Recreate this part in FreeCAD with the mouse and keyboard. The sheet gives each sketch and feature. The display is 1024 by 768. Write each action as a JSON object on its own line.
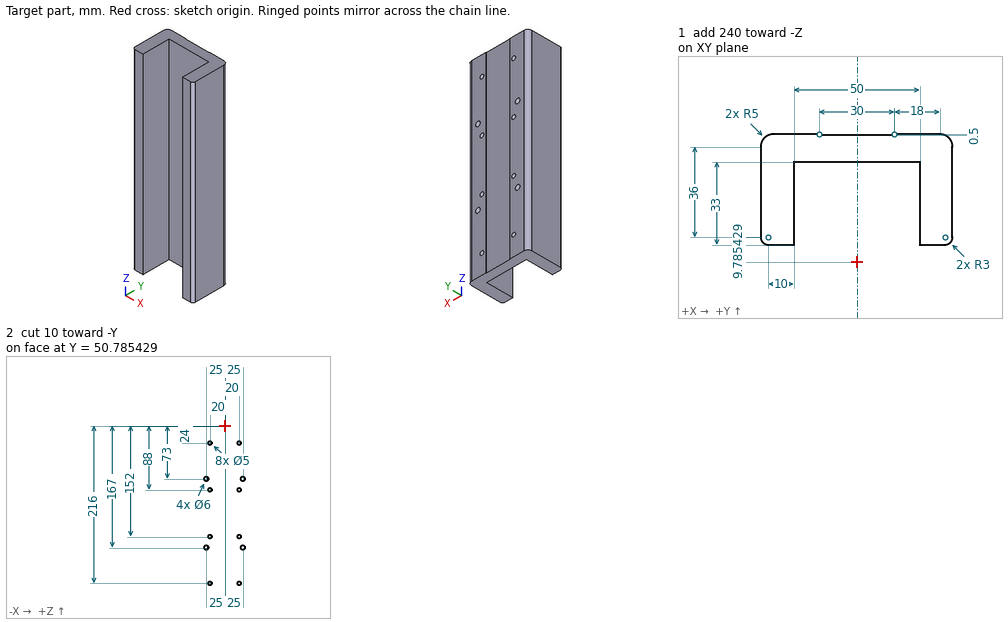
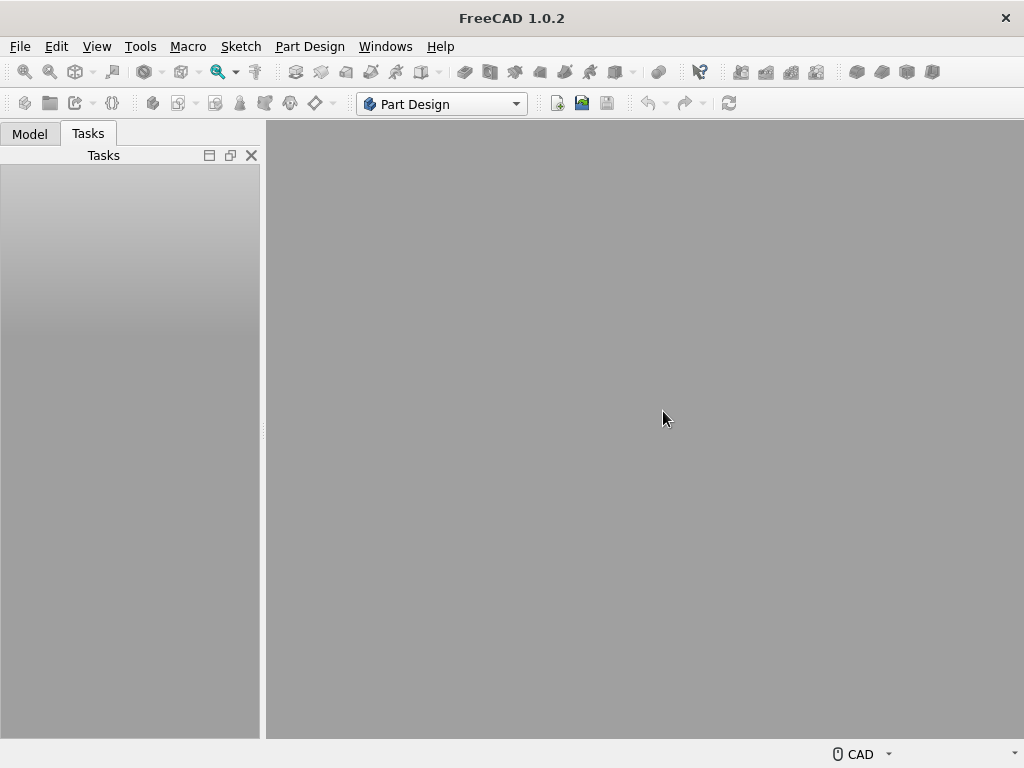
{"action": "left_click", "coordinate": [557, 104]}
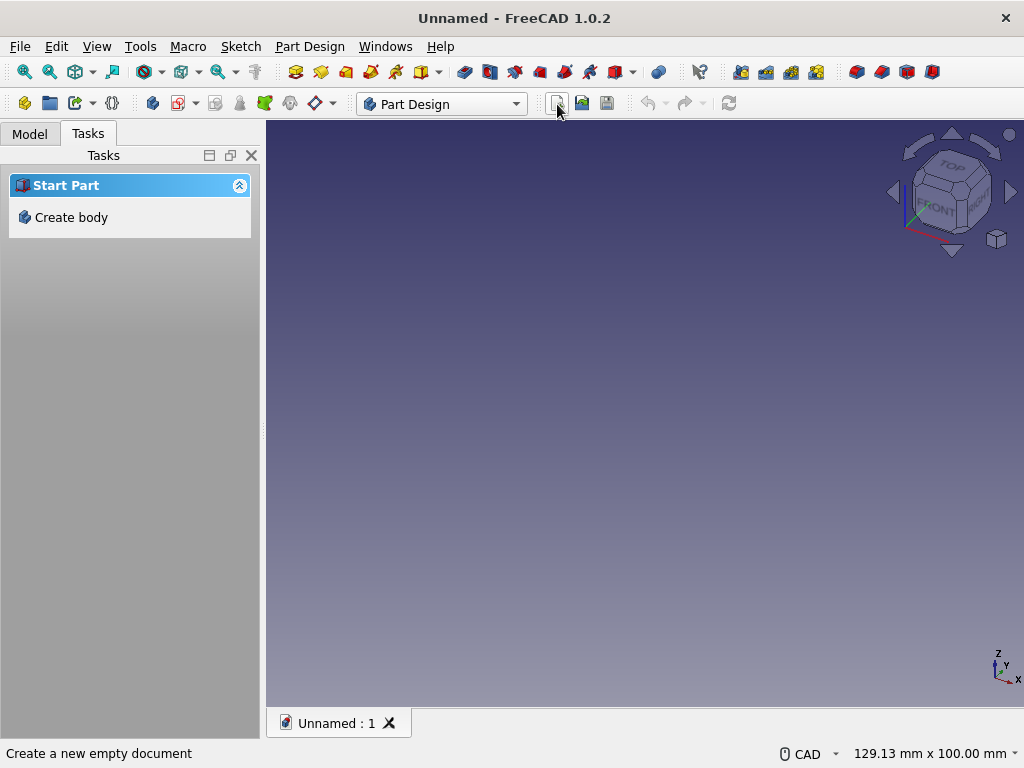
{"action": "left_click", "coordinate": [178, 104]}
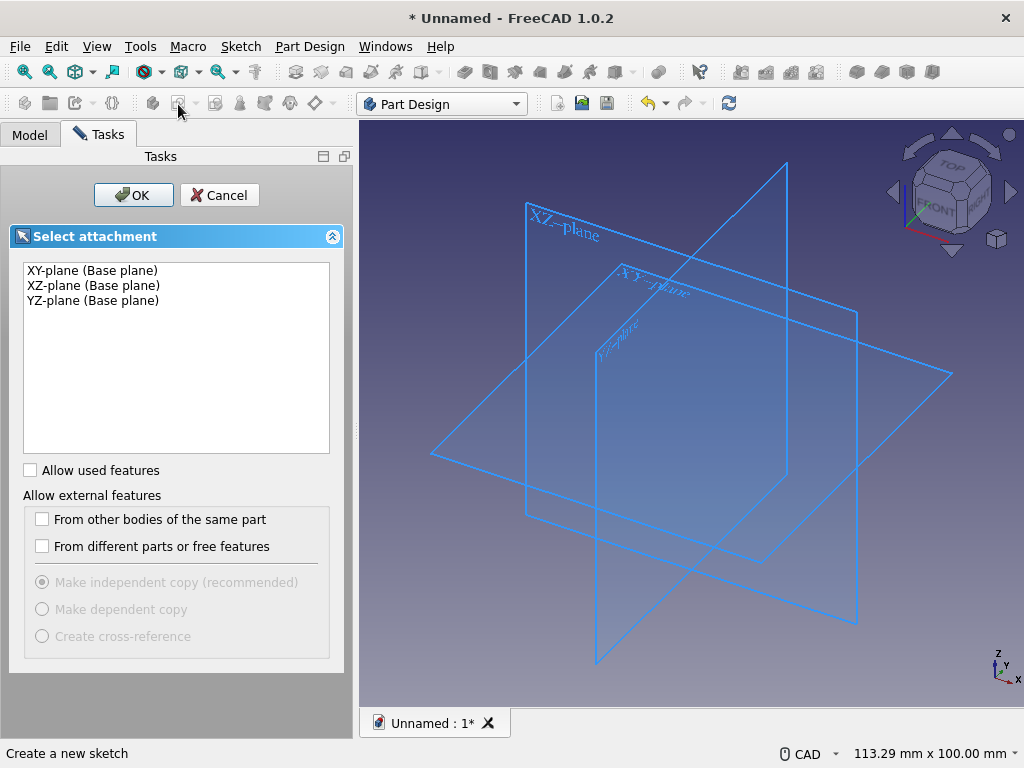
{"action": "left_click", "coordinate": [84, 270]}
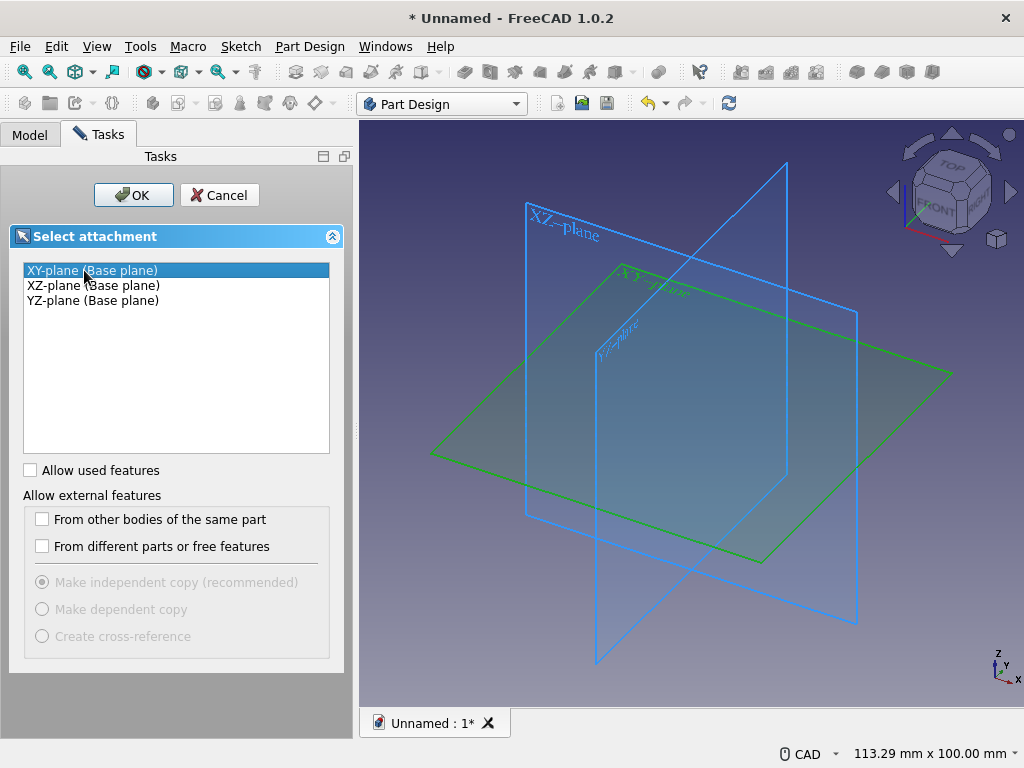
{"action": "left_click", "coordinate": [134, 195]}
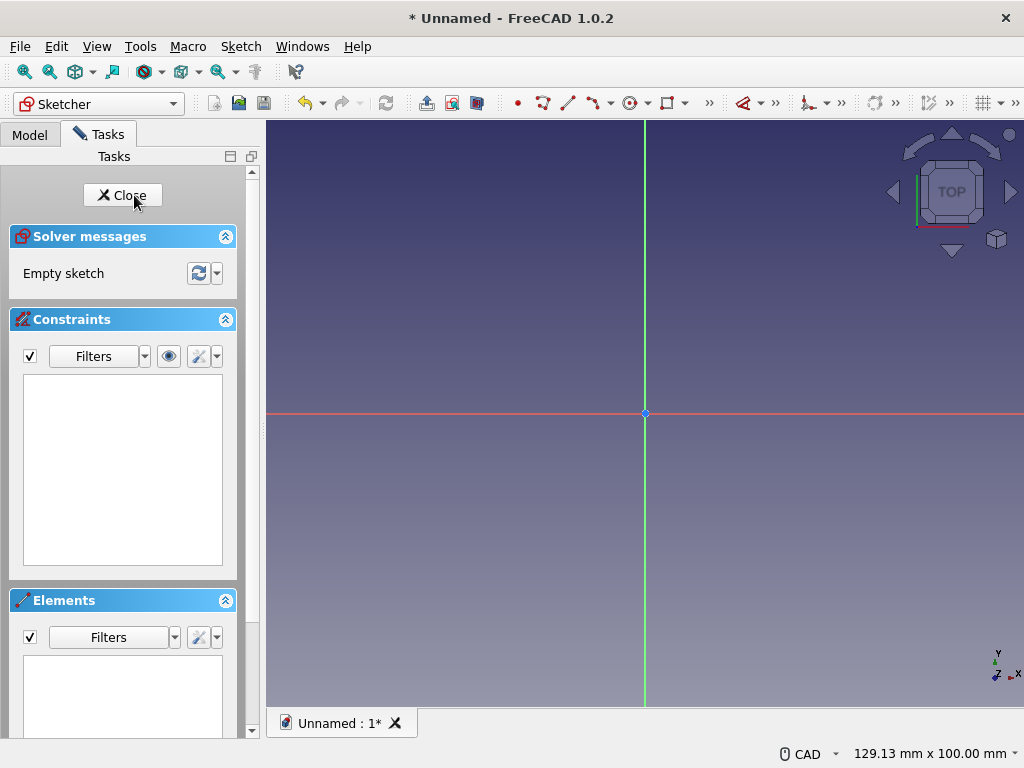
{"action": "scroll", "coordinate": [294, 679], "scroll_direction": "down", "scroll_amount": 1}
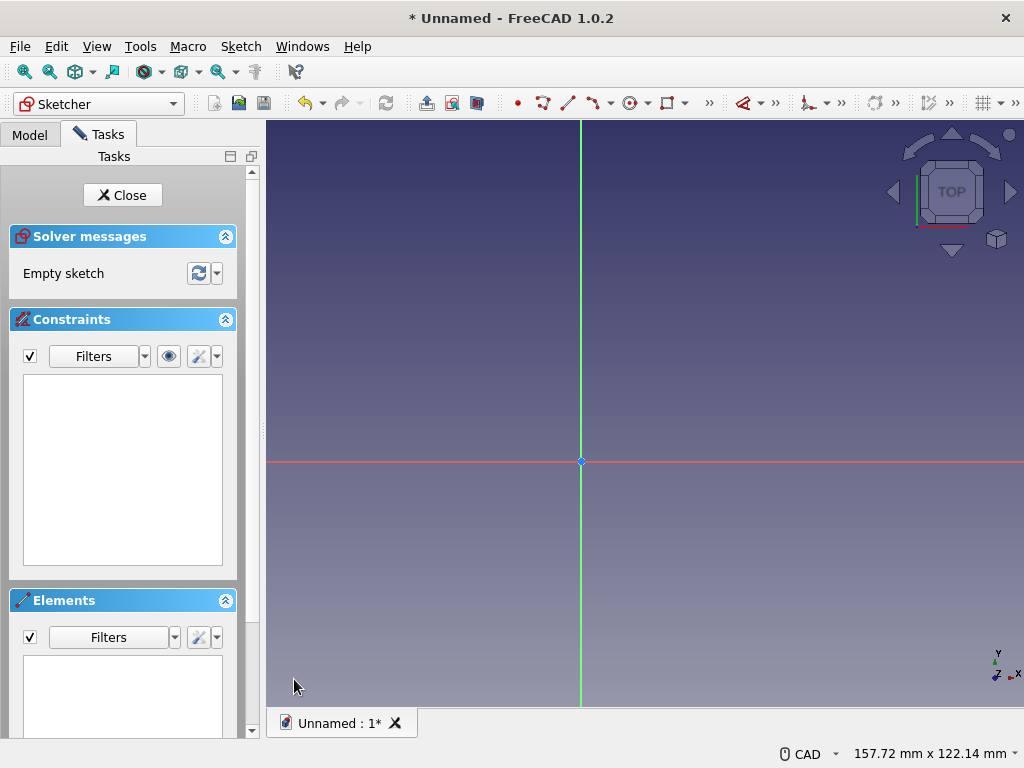
{"action": "left_click", "coordinate": [543, 104]}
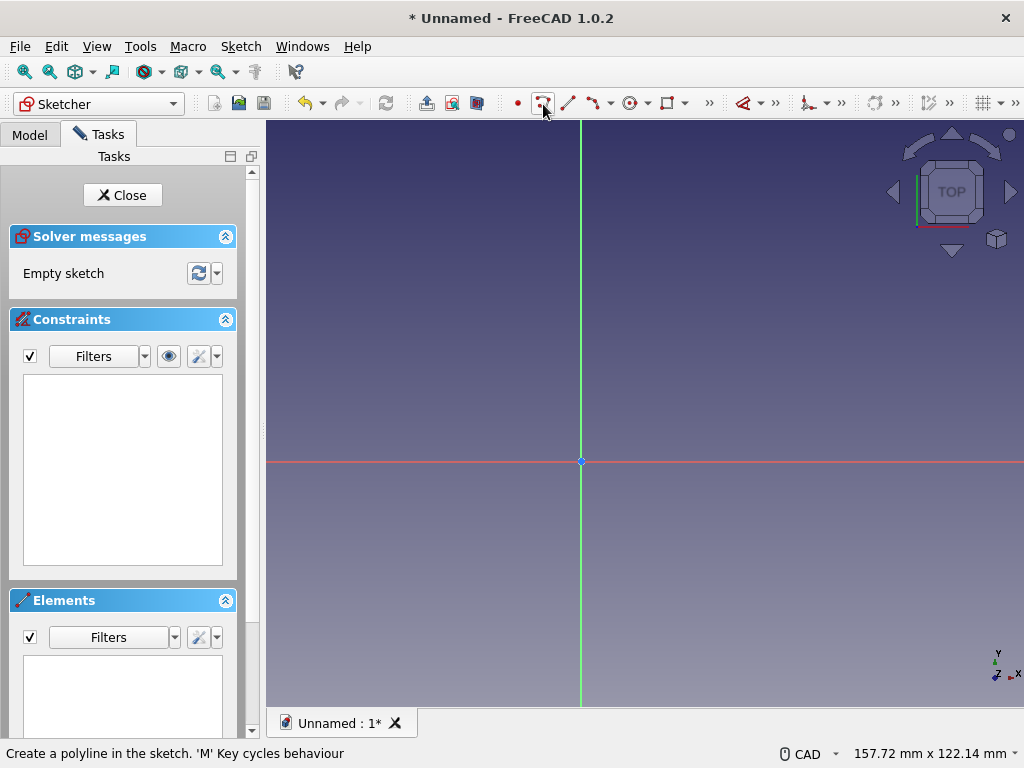
{"action": "left_click", "coordinate": [740, 218]}
{"action": "left_click", "coordinate": [653, 218]}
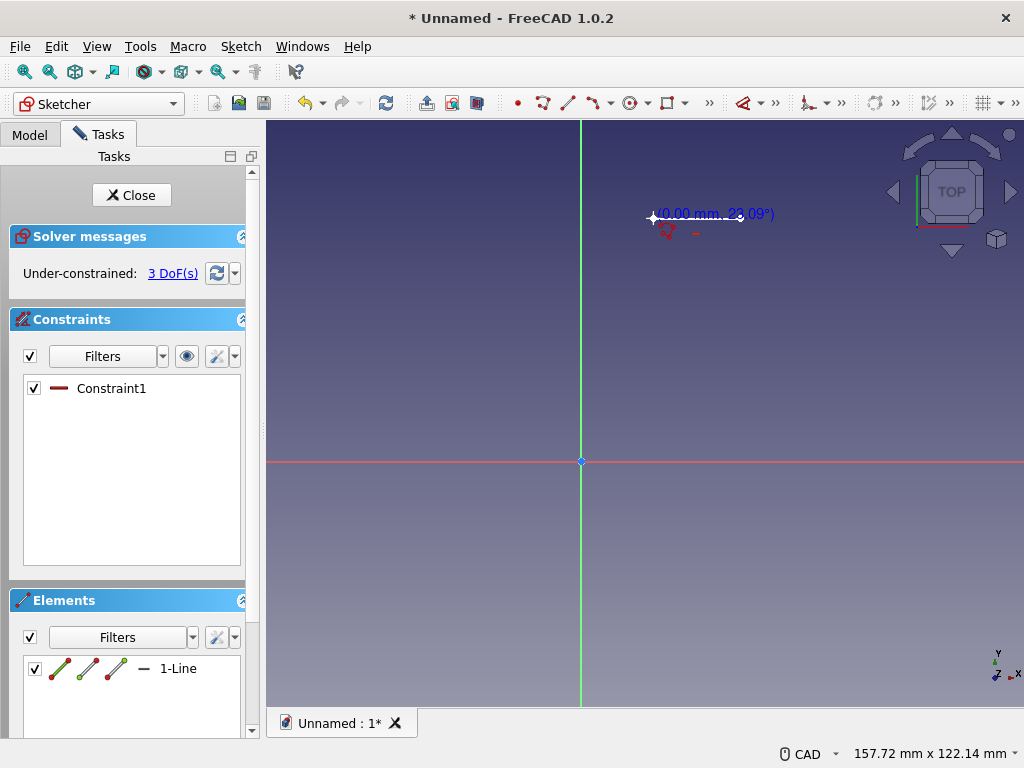
{"action": "scroll", "coordinate": [653, 220], "scroll_direction": "up", "scroll_amount": 10}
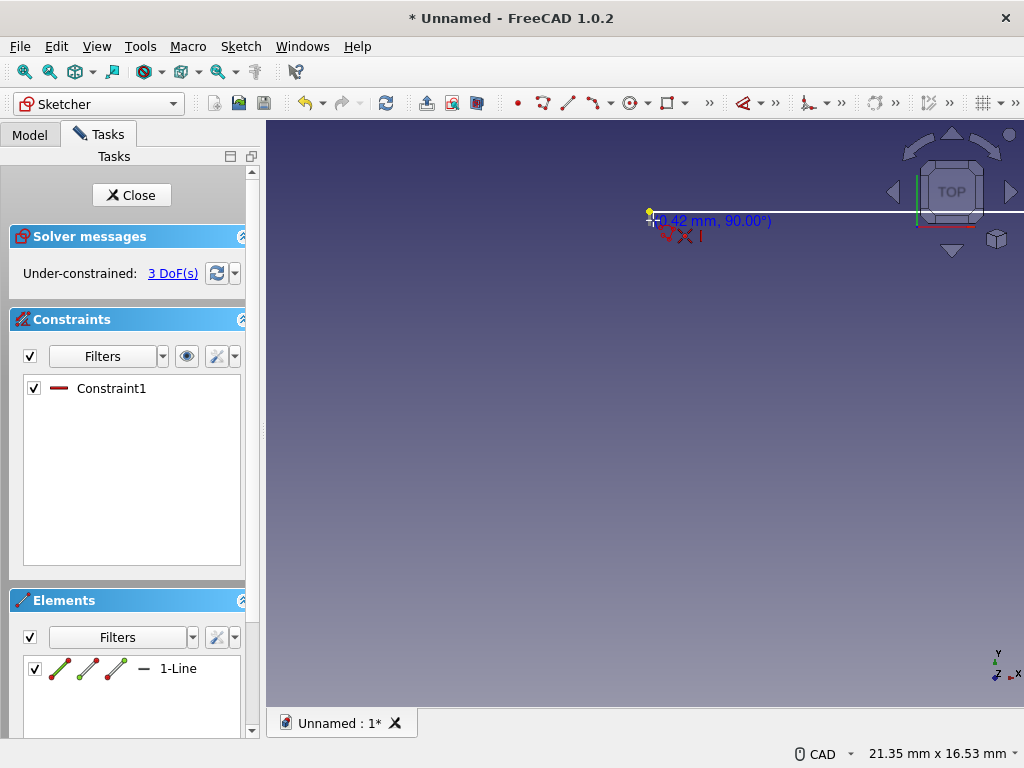
{"action": "left_click", "coordinate": [650, 220]}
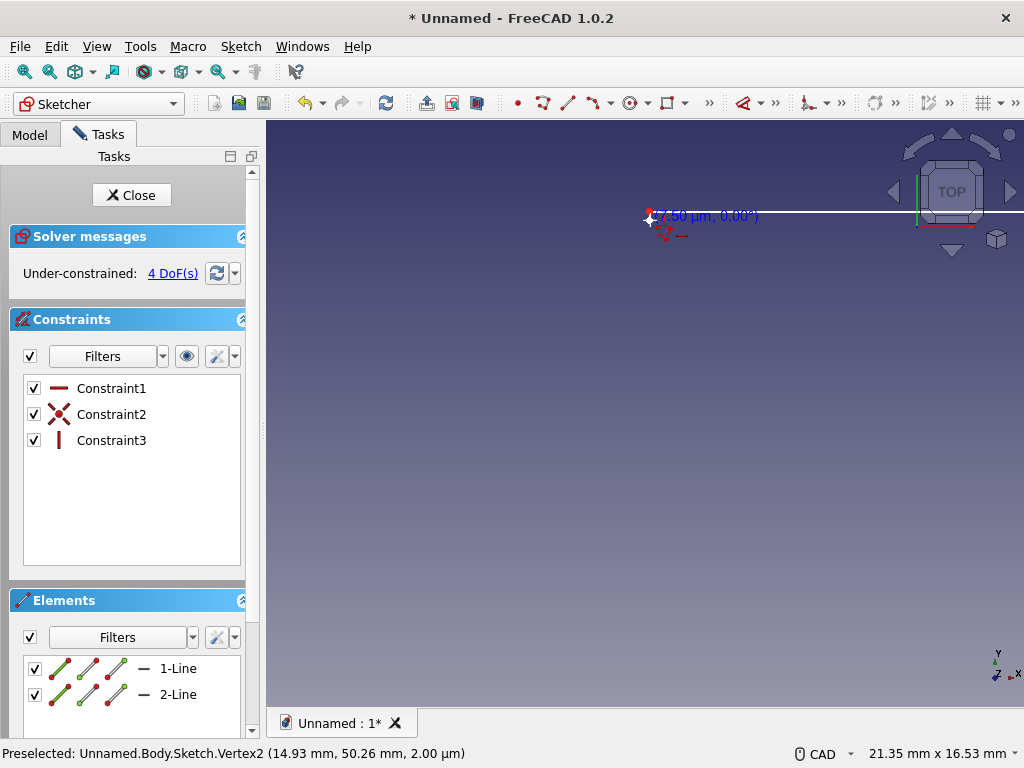
{"action": "scroll", "coordinate": [648, 305], "scroll_direction": "down", "scroll_amount": 10}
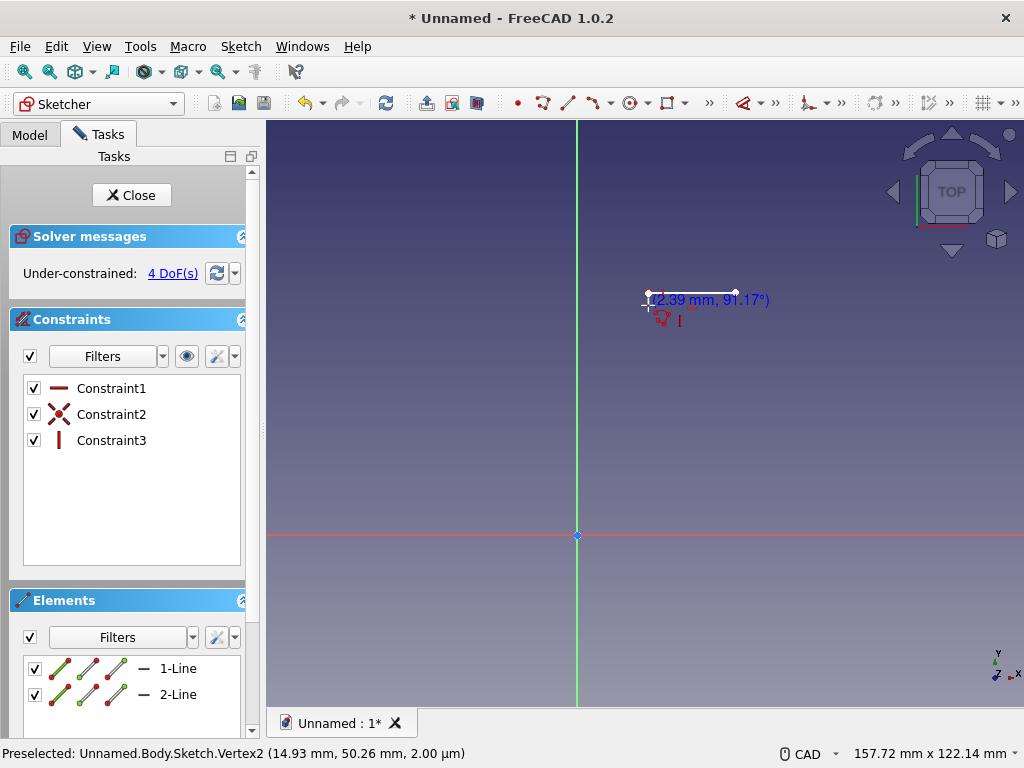
{"action": "left_click", "coordinate": [505, 294]}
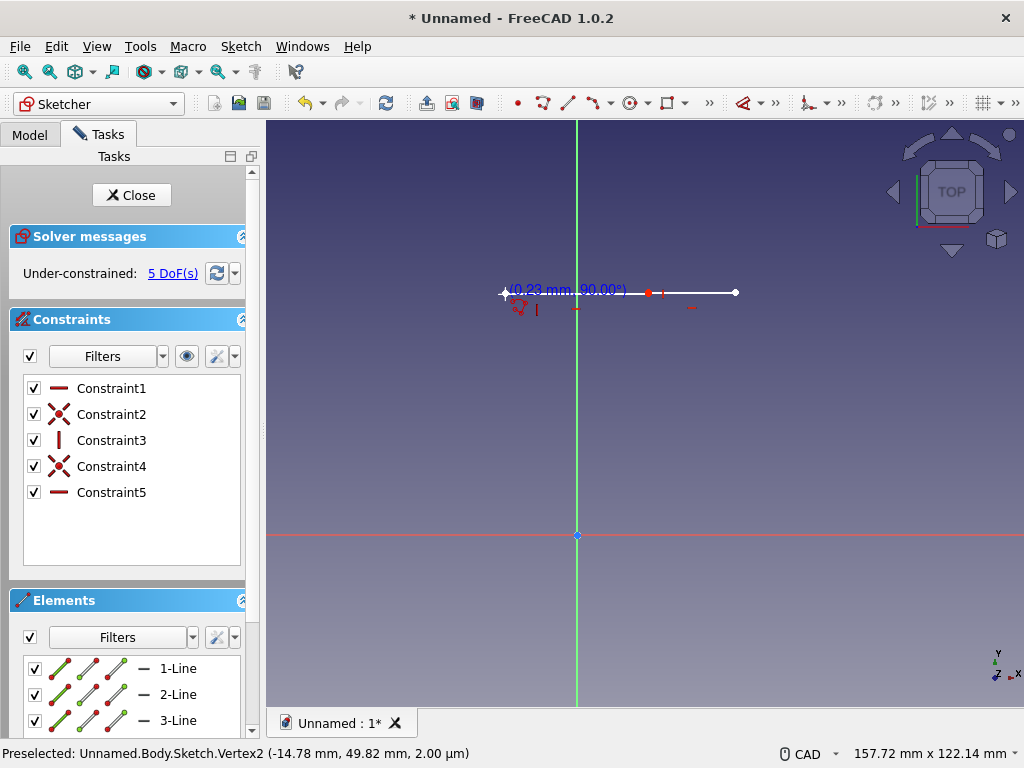
{"action": "scroll", "coordinate": [505, 291], "scroll_direction": "up", "scroll_amount": 10}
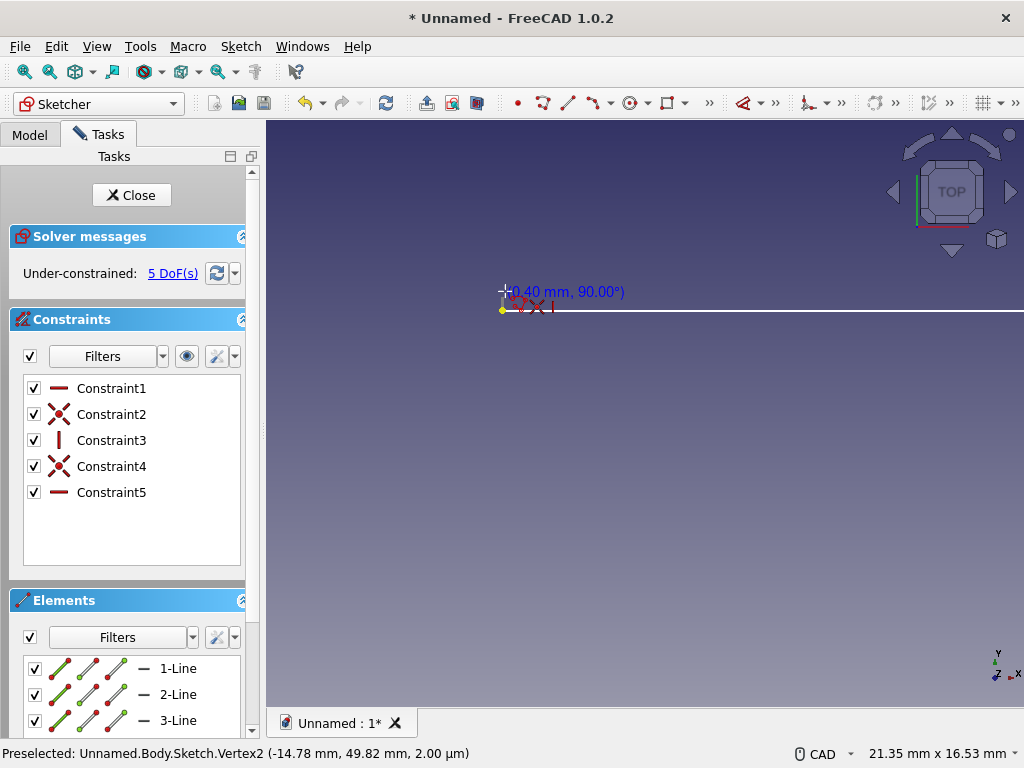
{"action": "left_click", "coordinate": [503, 292]}